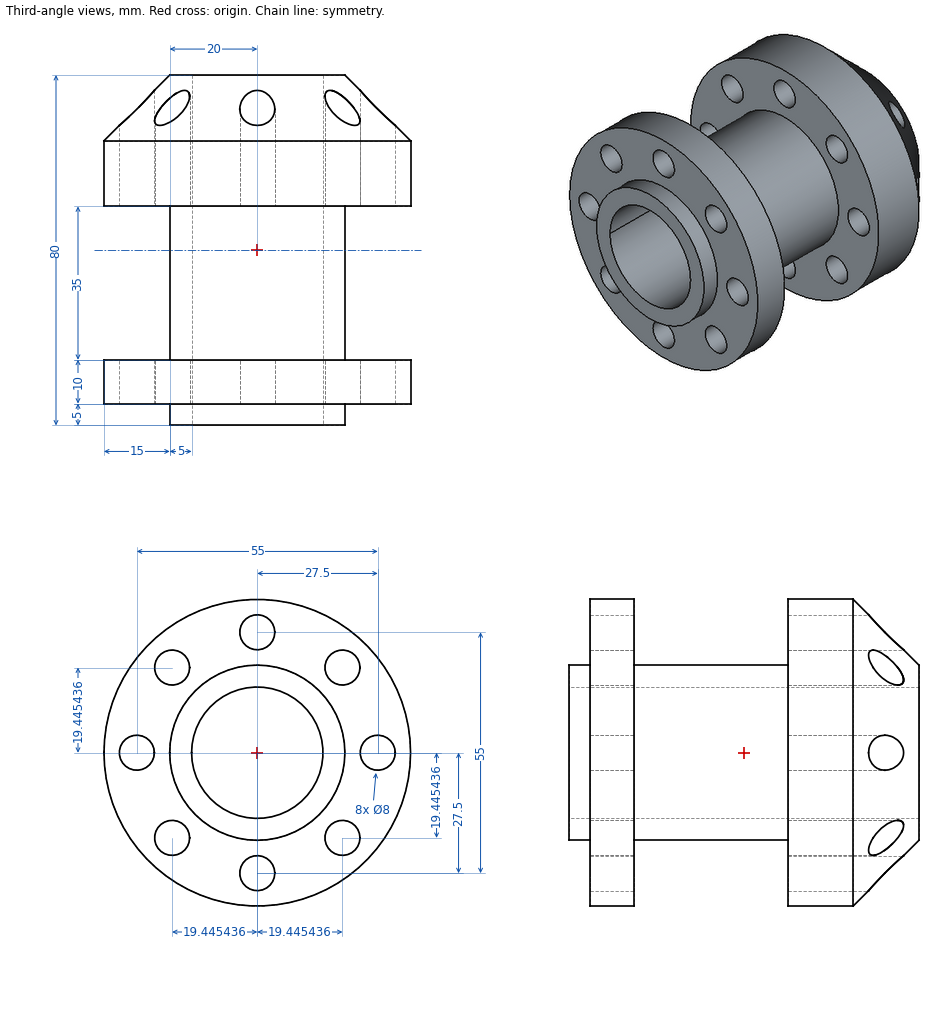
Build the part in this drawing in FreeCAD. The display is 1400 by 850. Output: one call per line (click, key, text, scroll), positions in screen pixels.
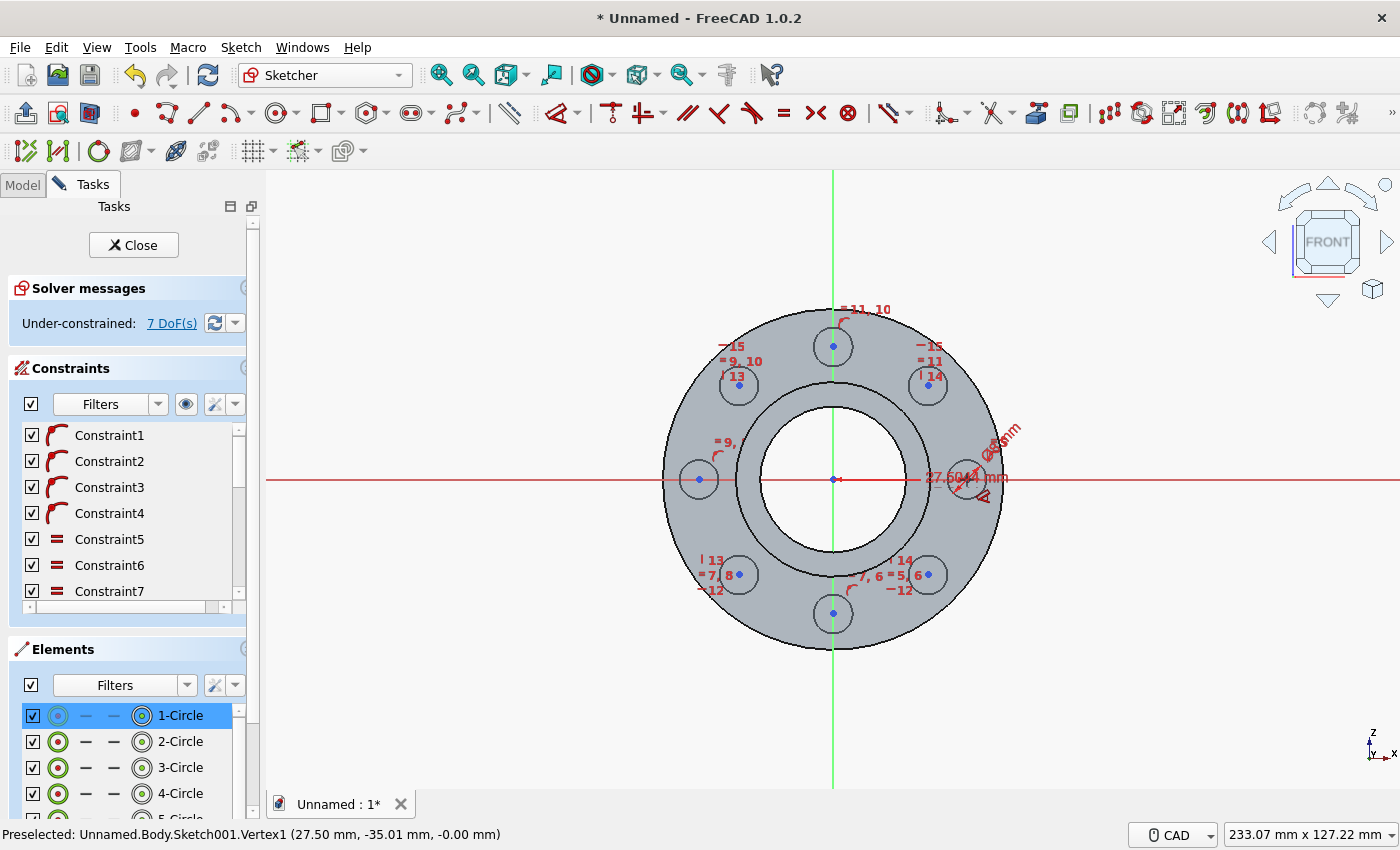
click(699, 480)
click(771, 514)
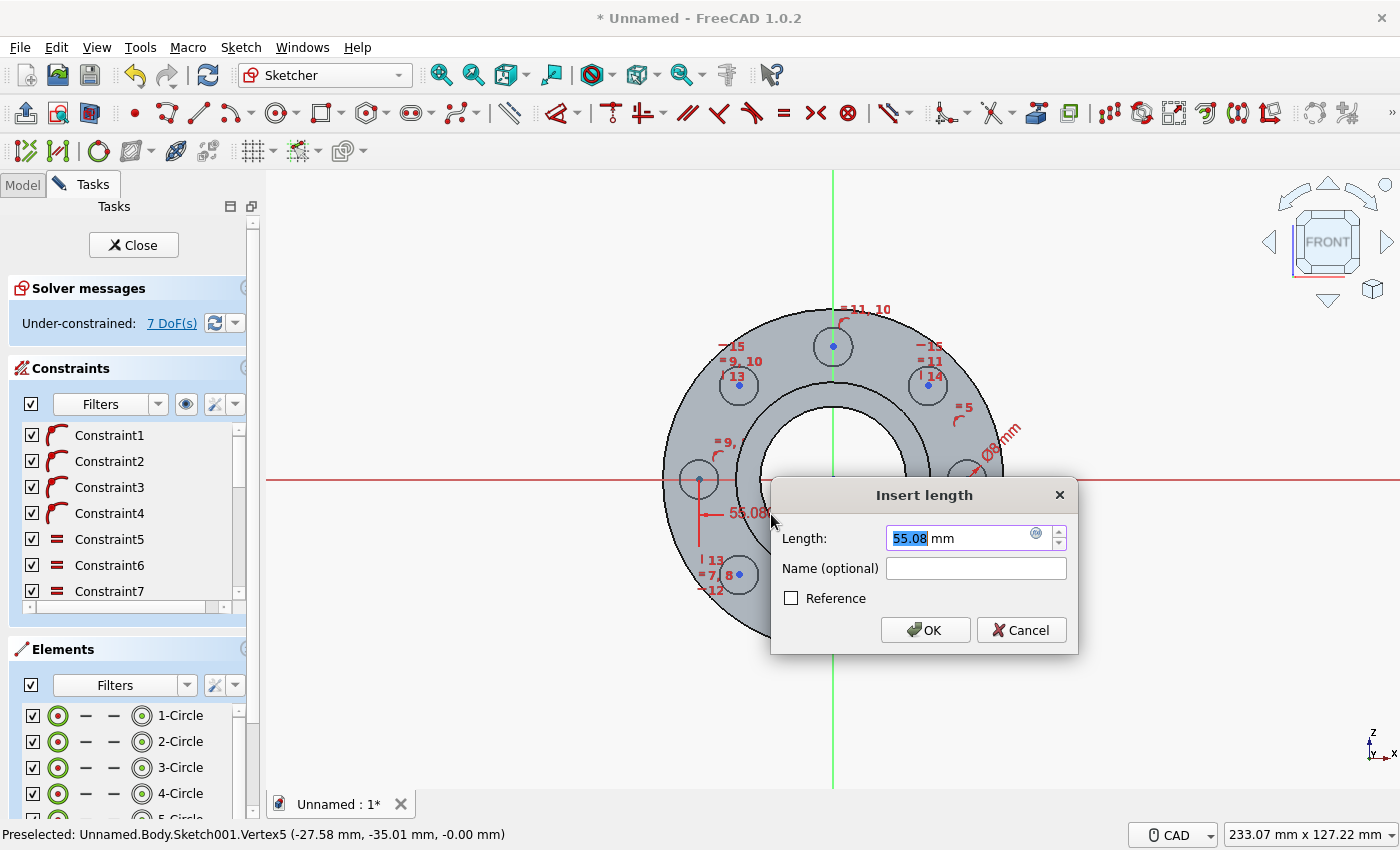
text(55)
key(Return)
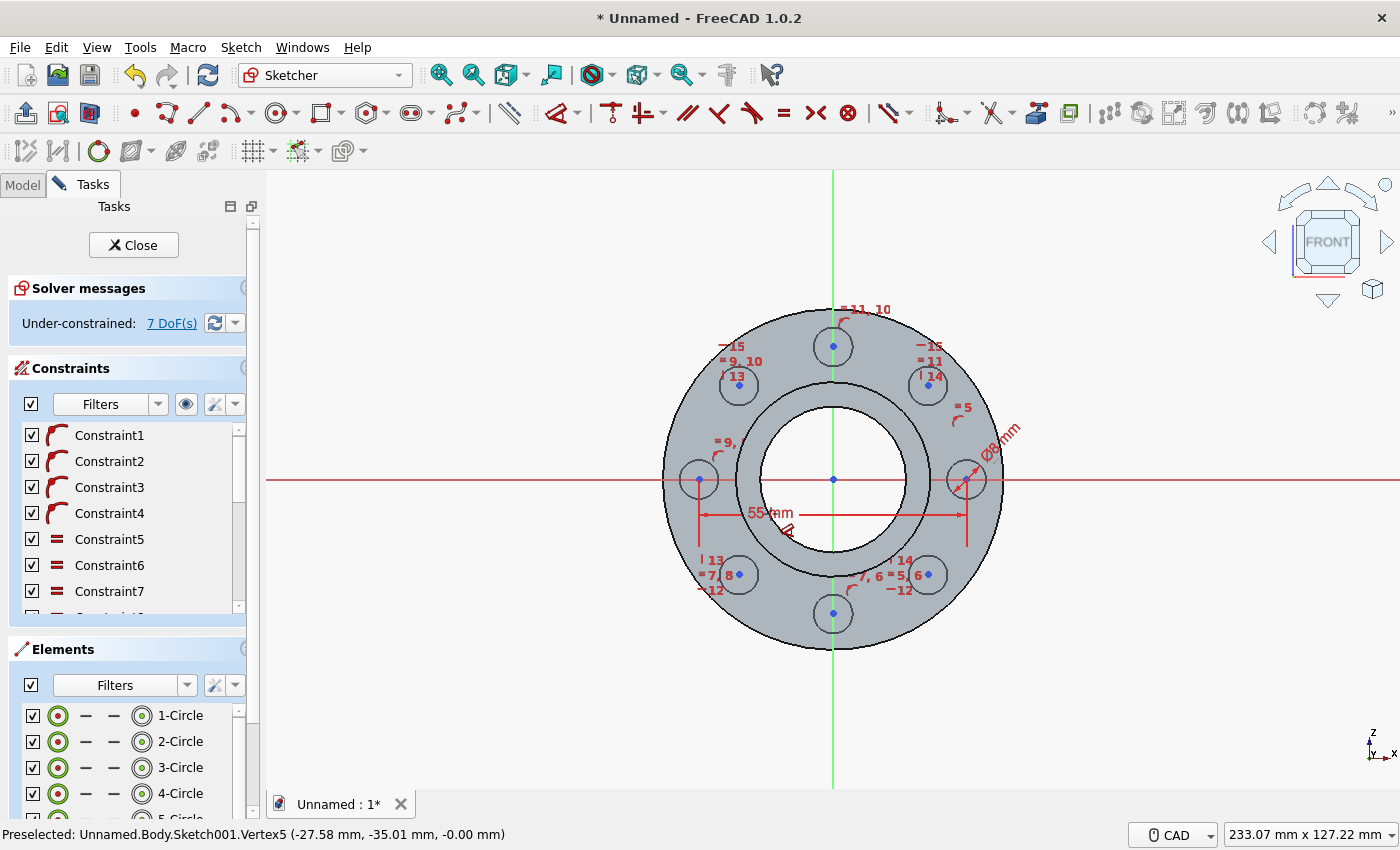
click(833, 614)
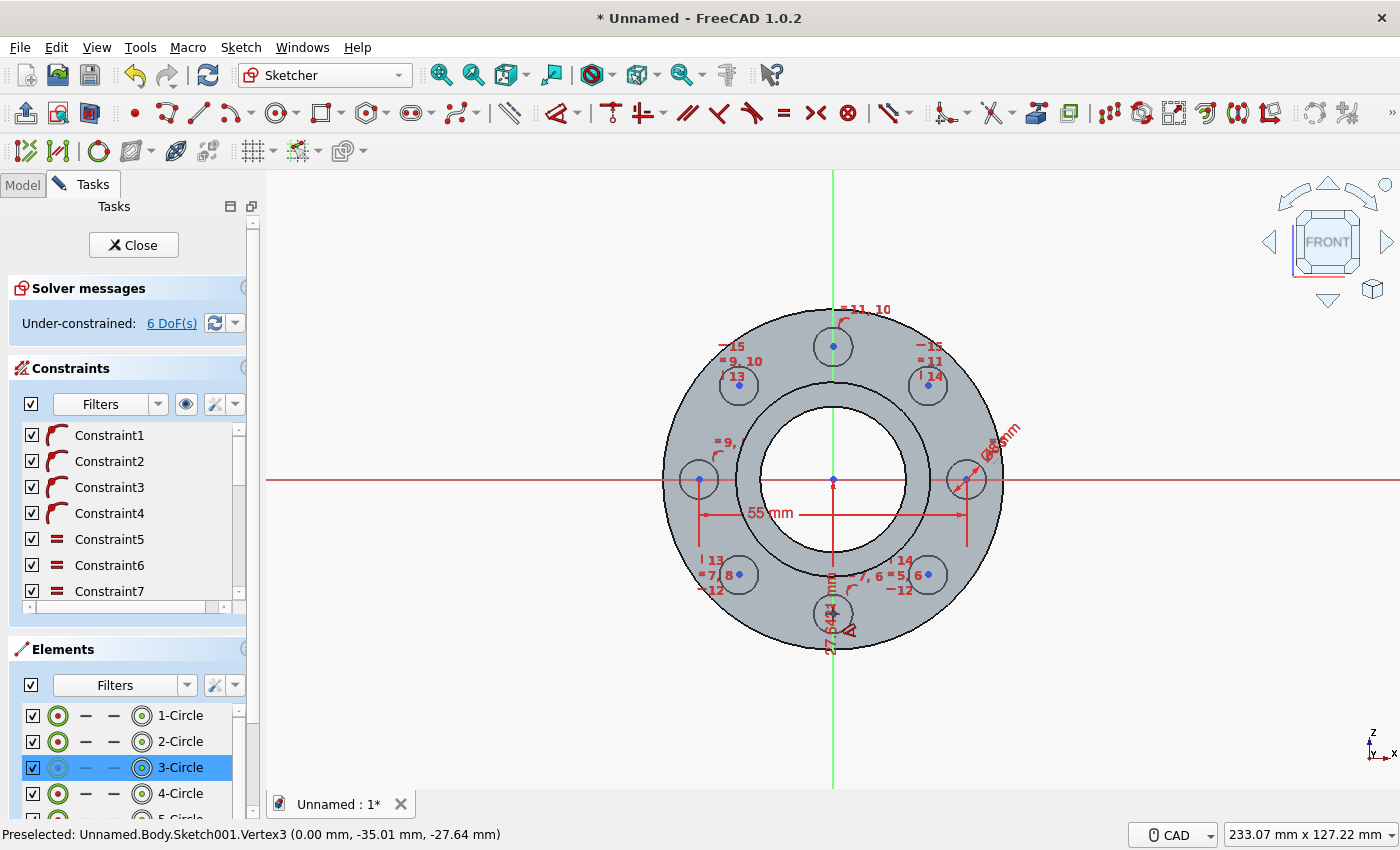
click(833, 347)
click(867, 419)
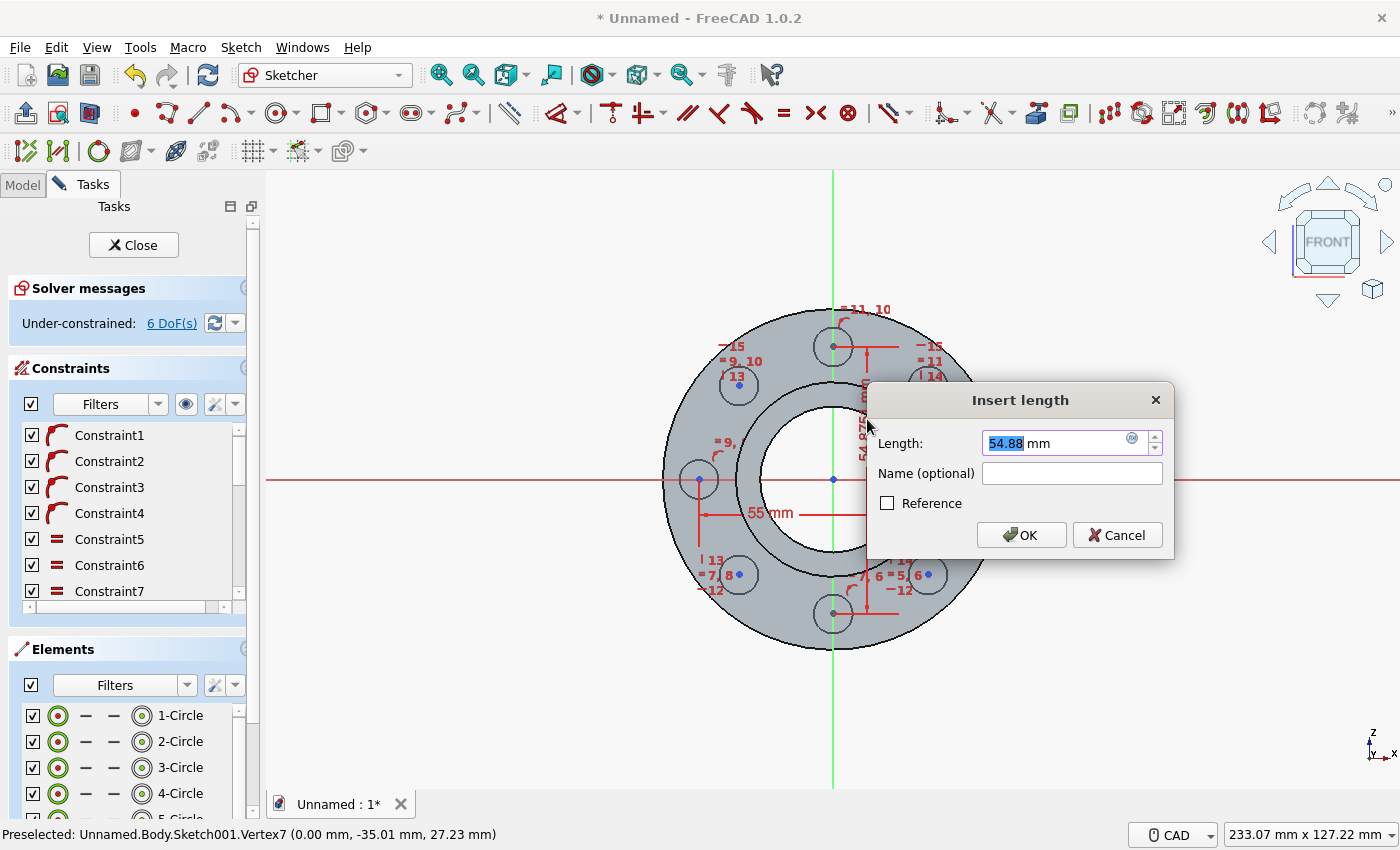
text(55)
key(Return)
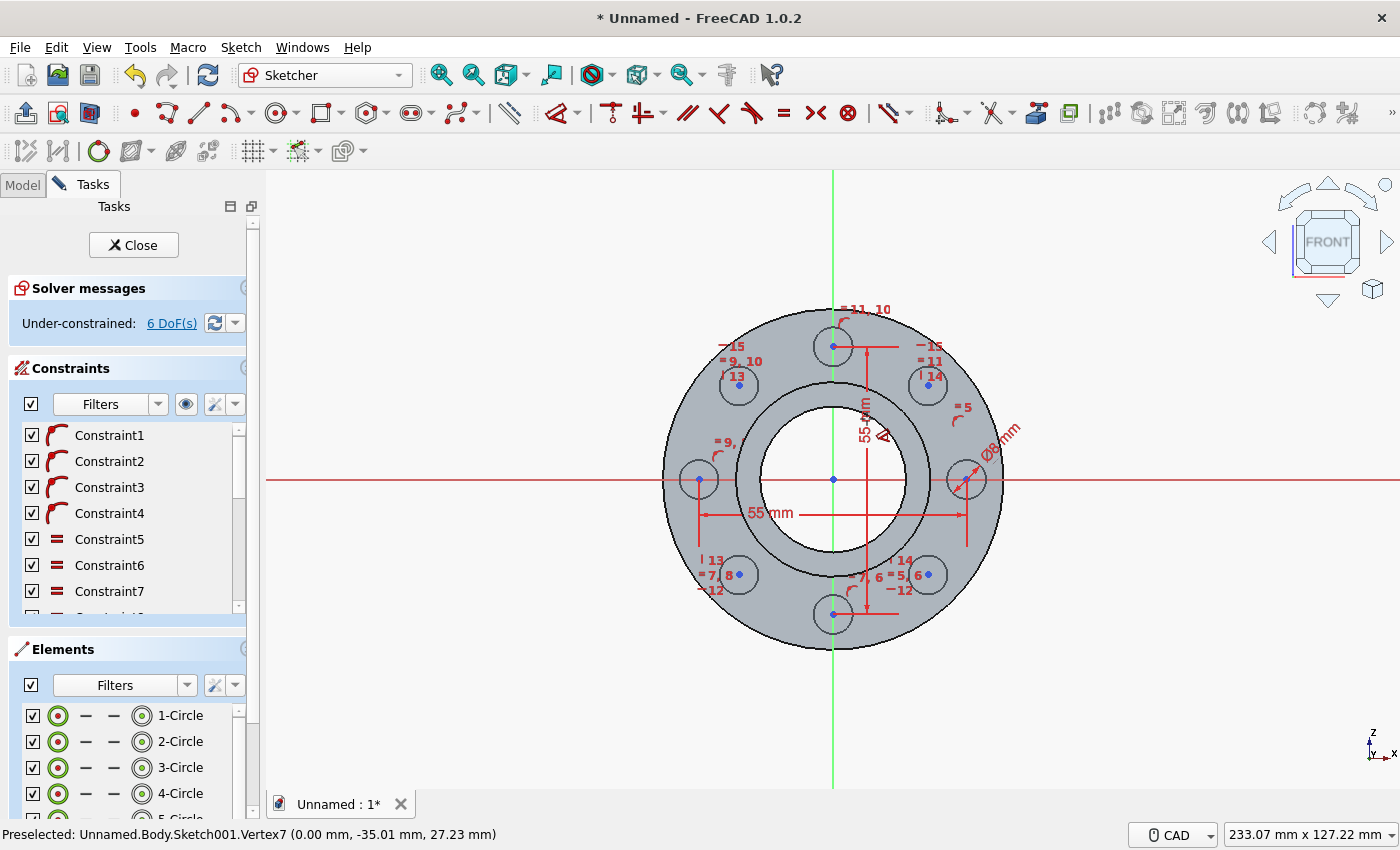
click(967, 480)
click(900, 514)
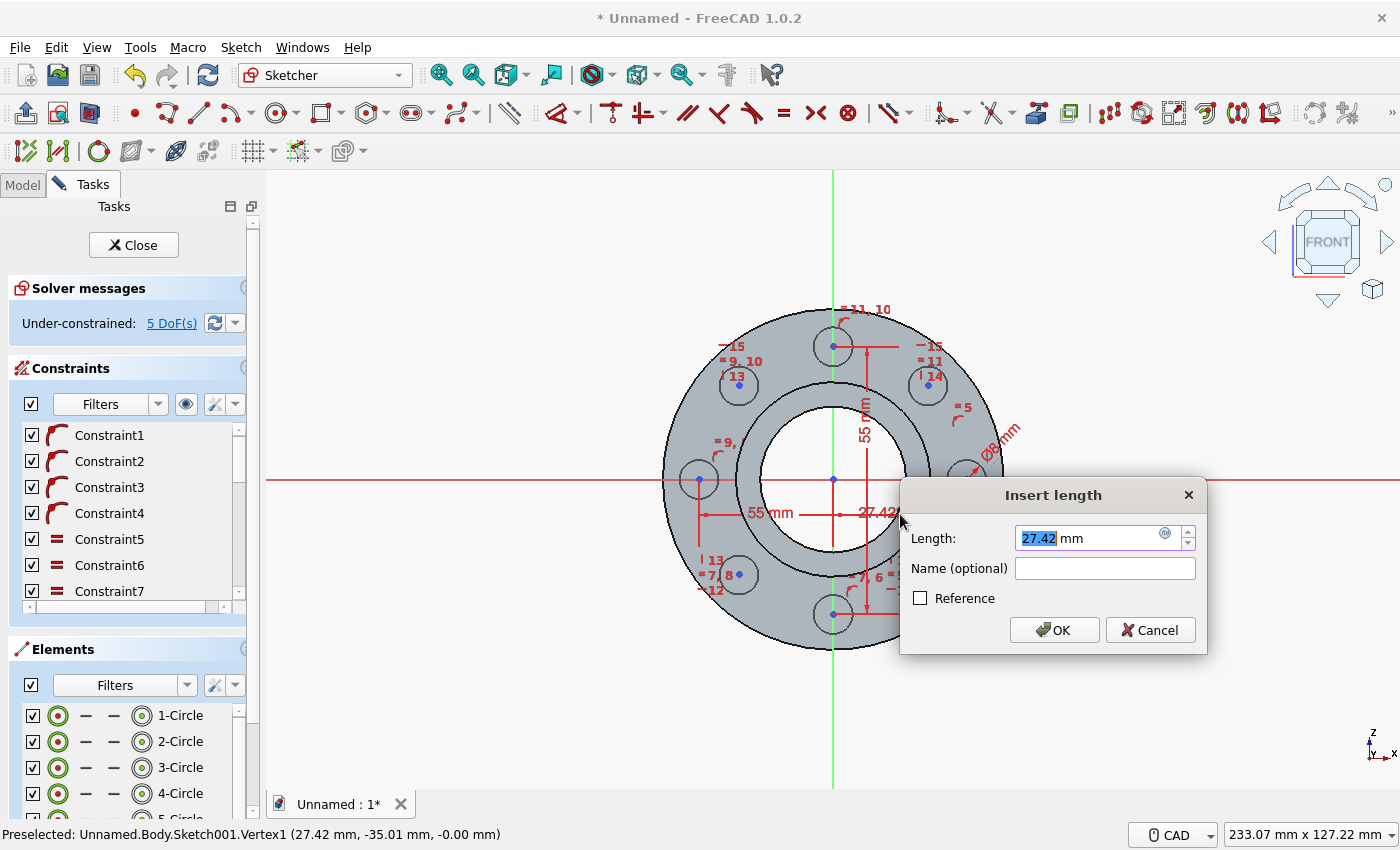
text(27.5)
key(Return)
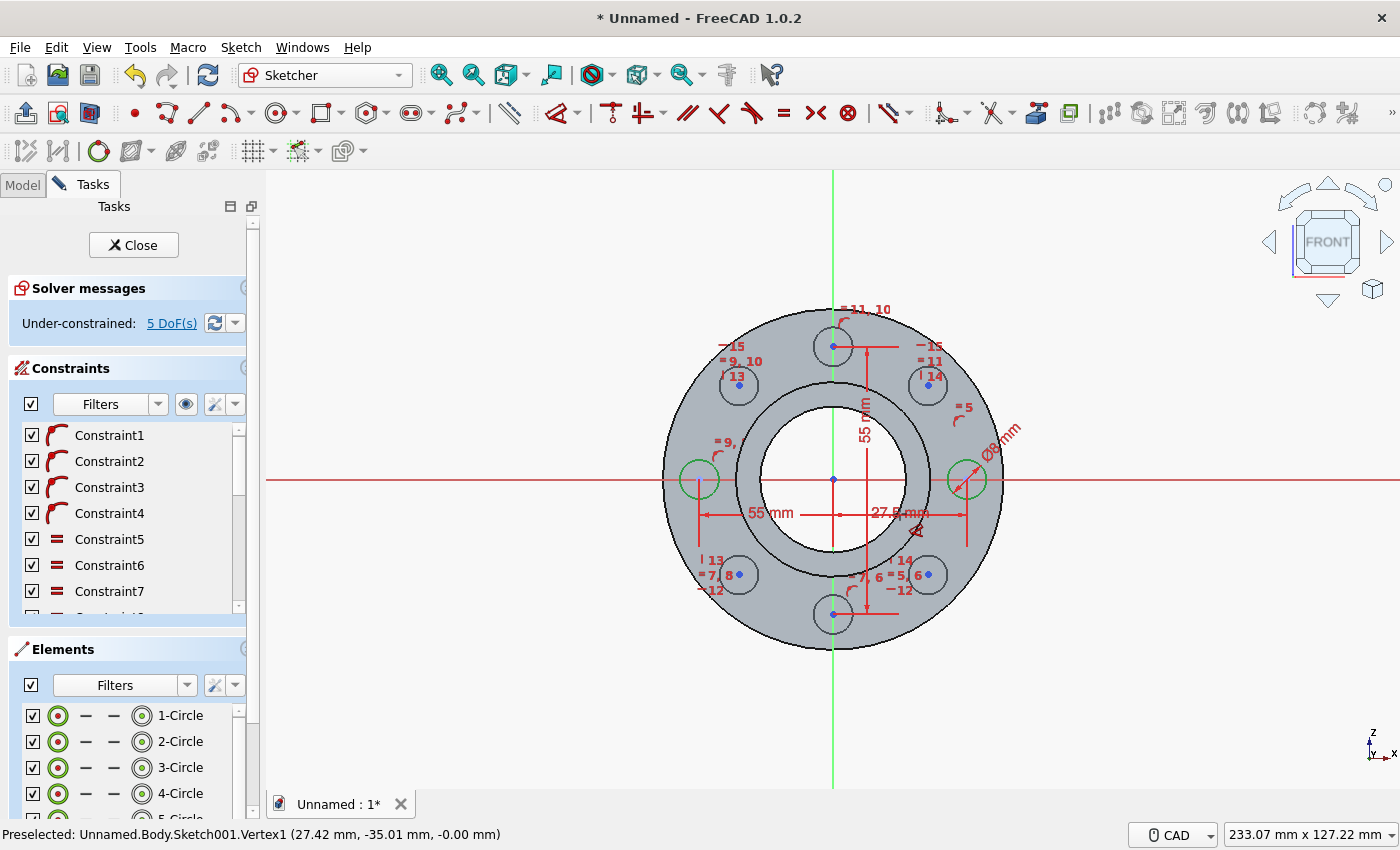
click(833, 614)
click(867, 547)